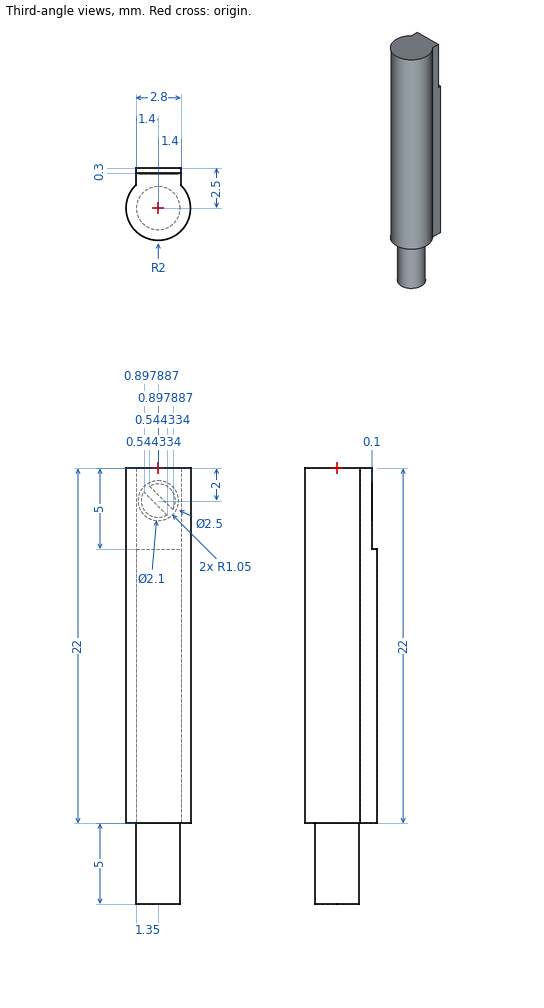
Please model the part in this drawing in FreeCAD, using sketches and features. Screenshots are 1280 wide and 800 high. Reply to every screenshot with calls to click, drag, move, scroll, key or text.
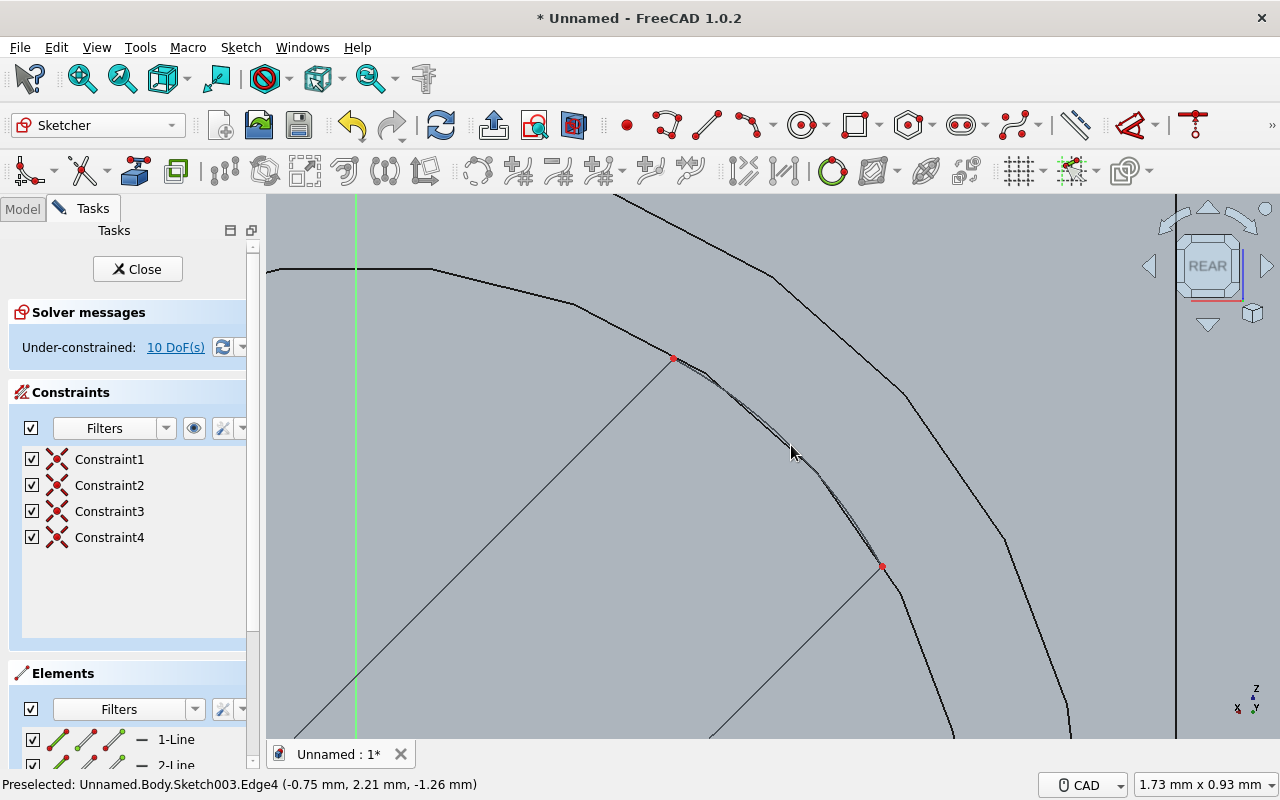
scroll(793, 444, down, 8)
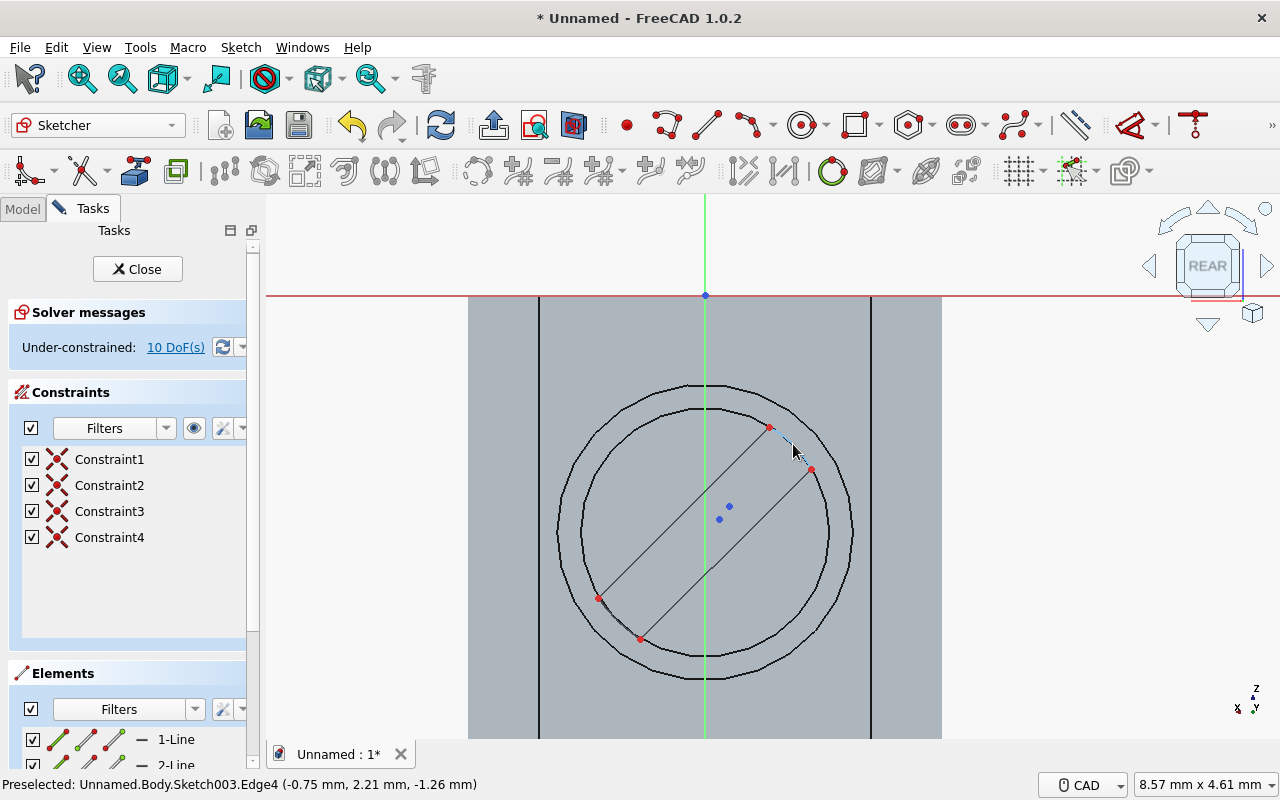
click(609, 612)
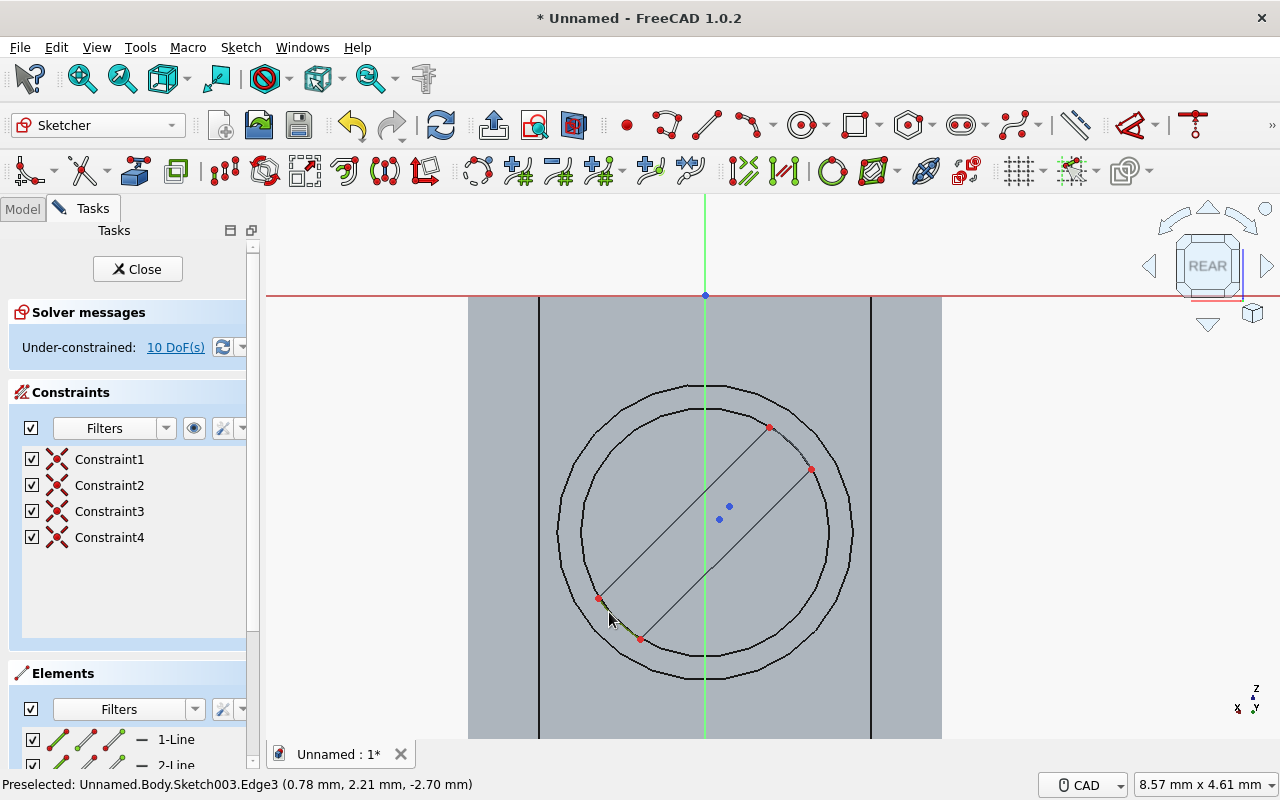
click(801, 454)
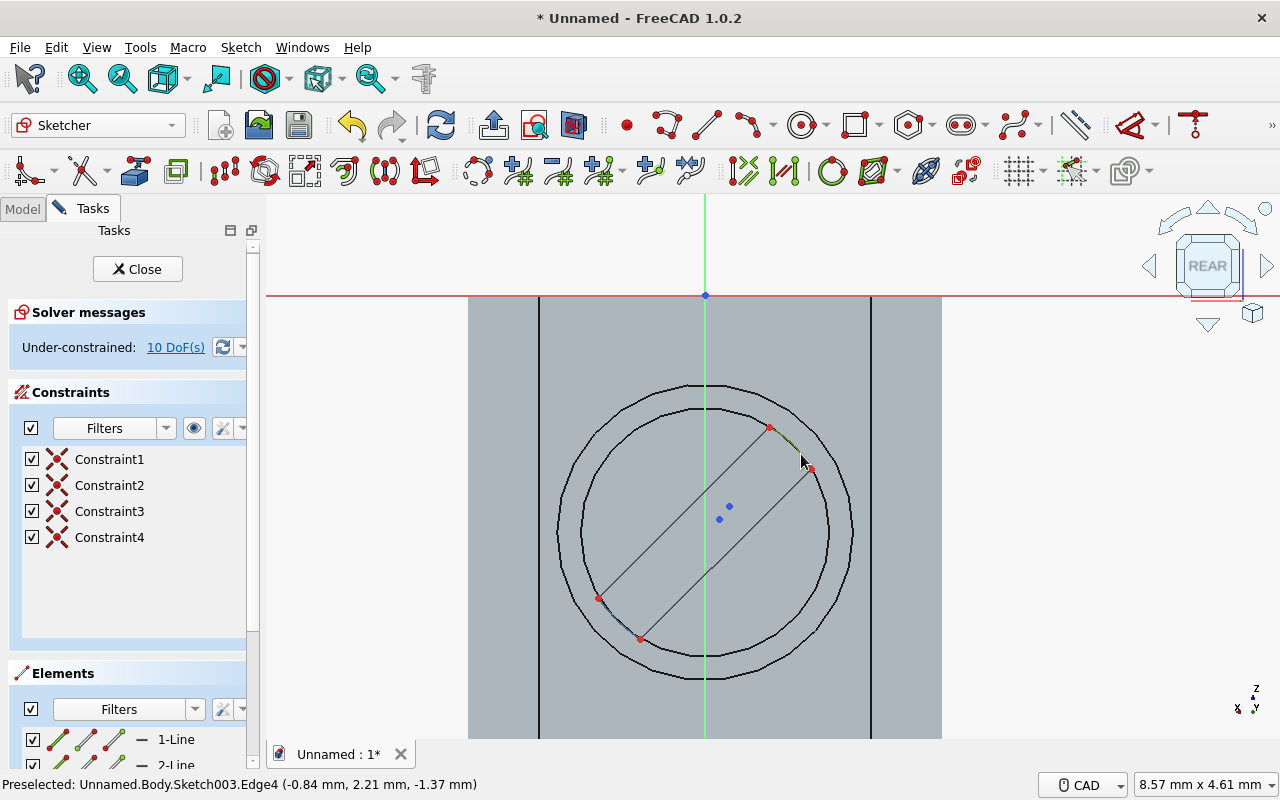
click(1194, 126)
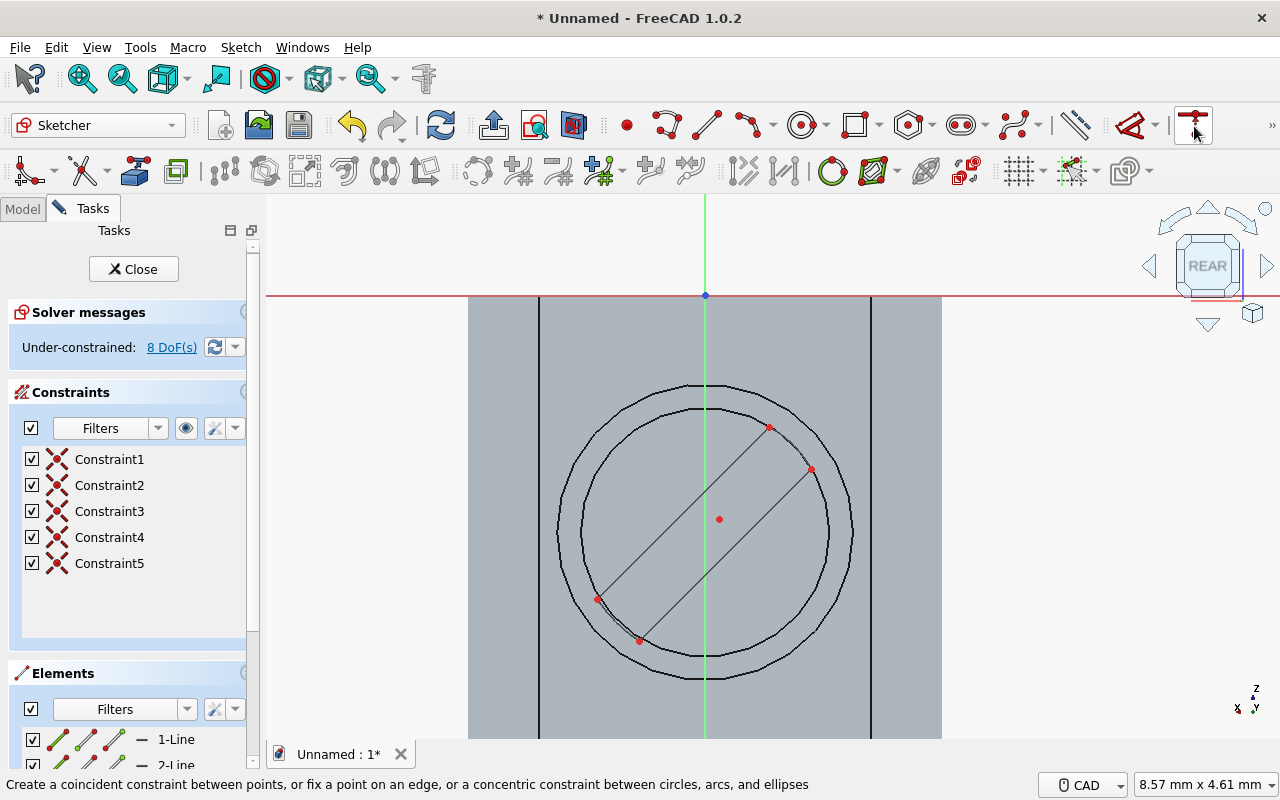
click(608, 614)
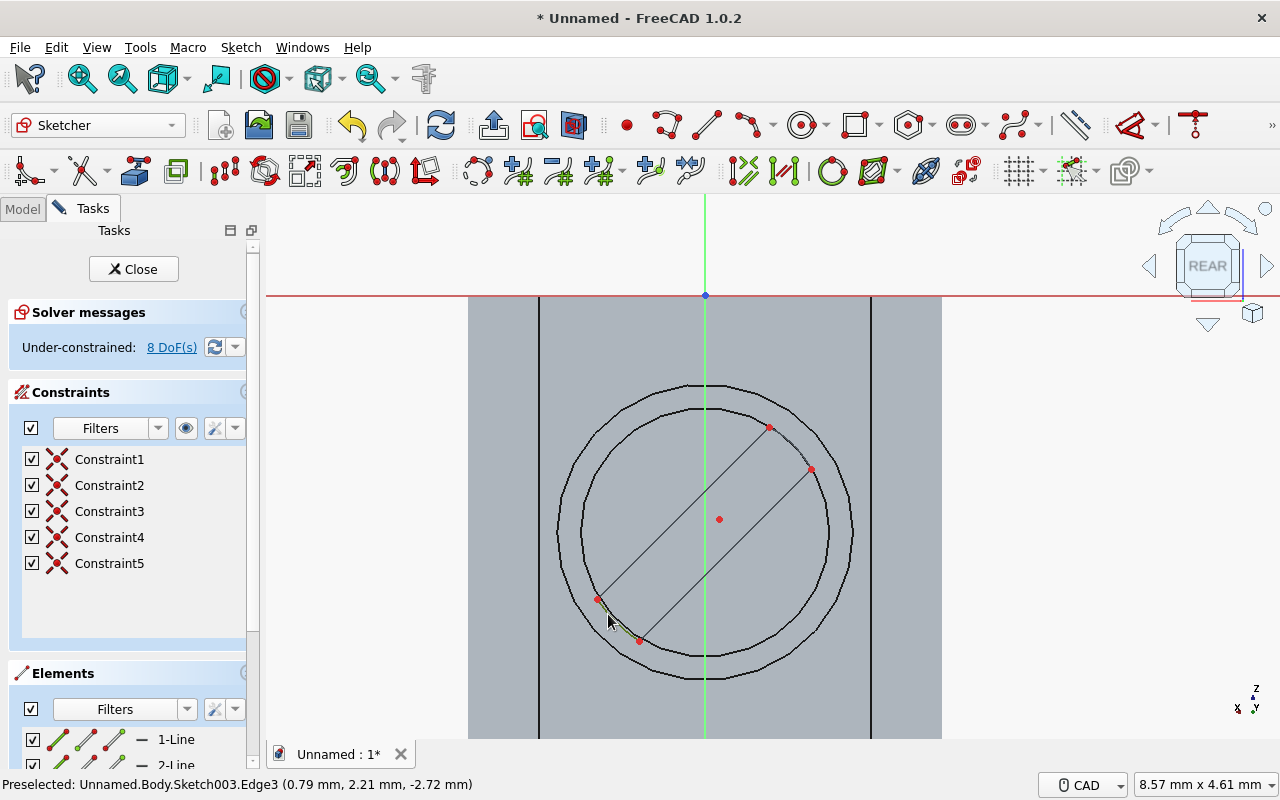
click(801, 454)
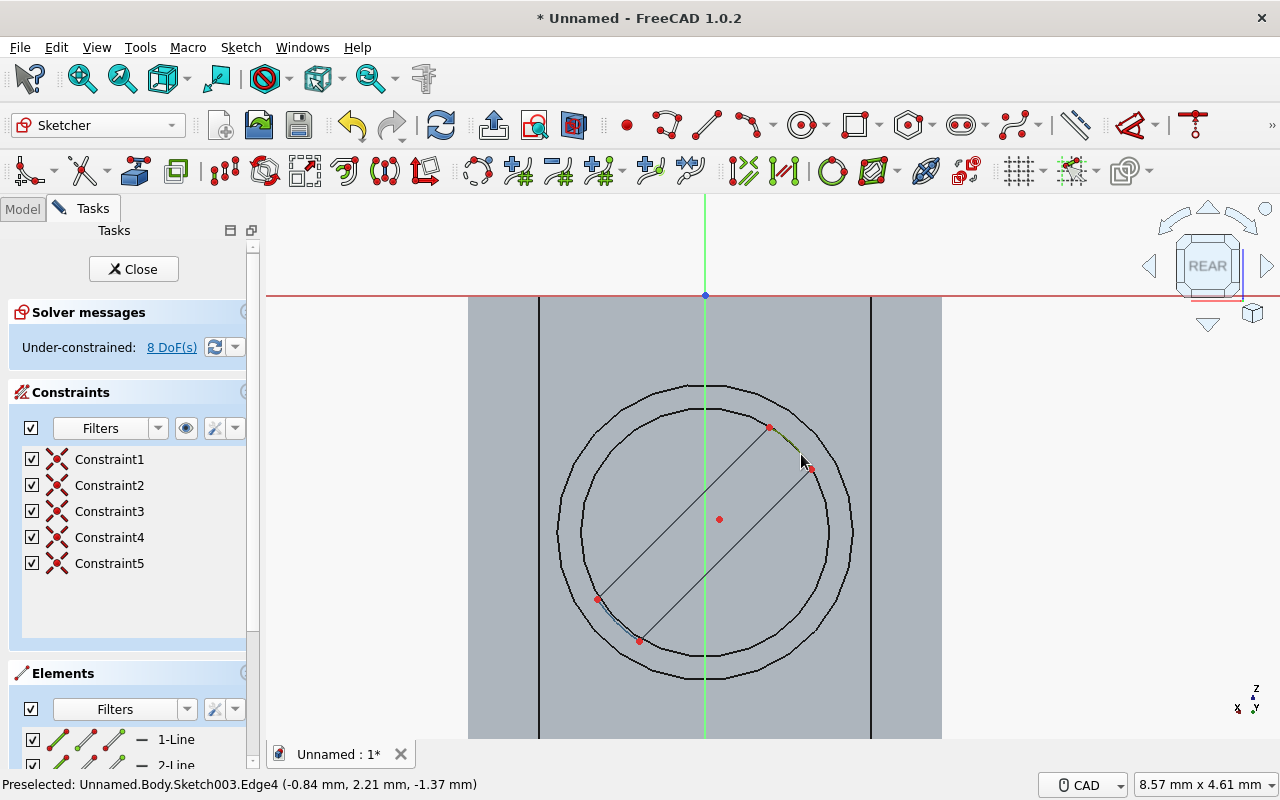
key(e)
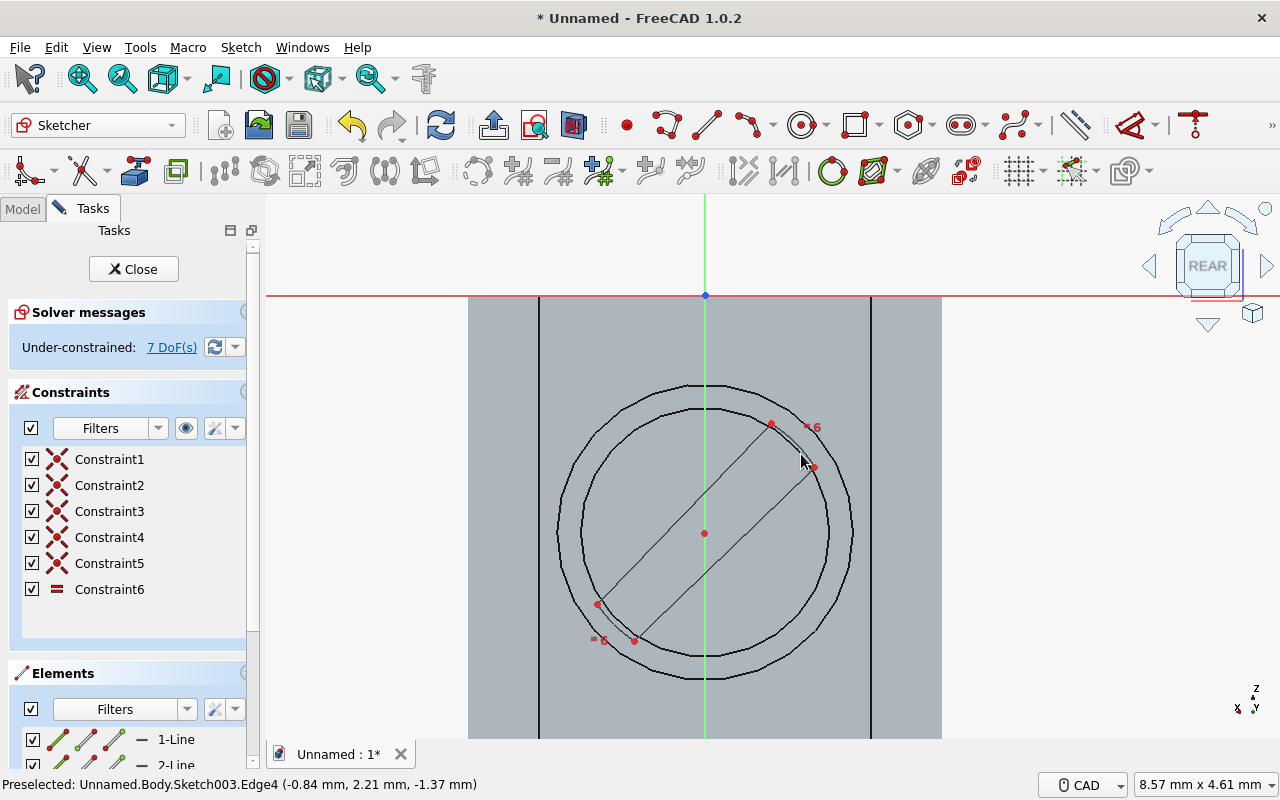
click(705, 534)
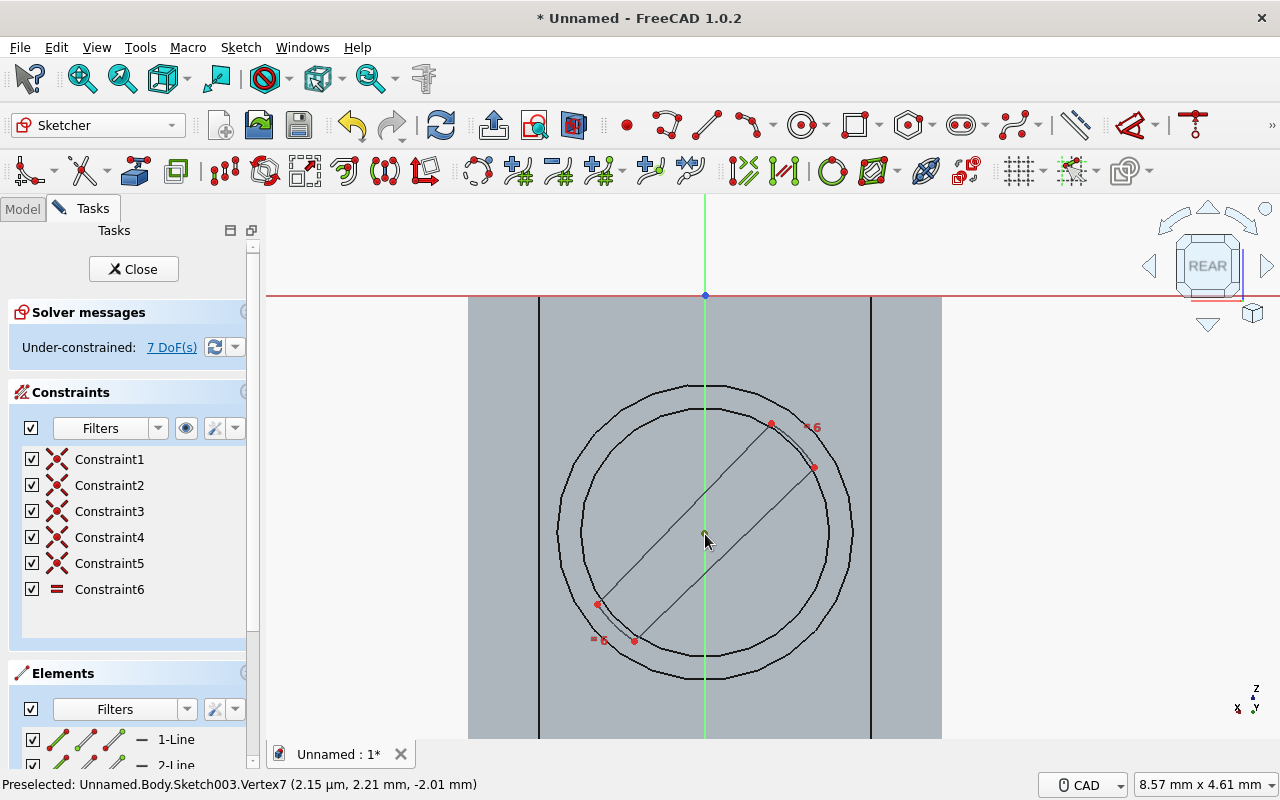
click(705, 676)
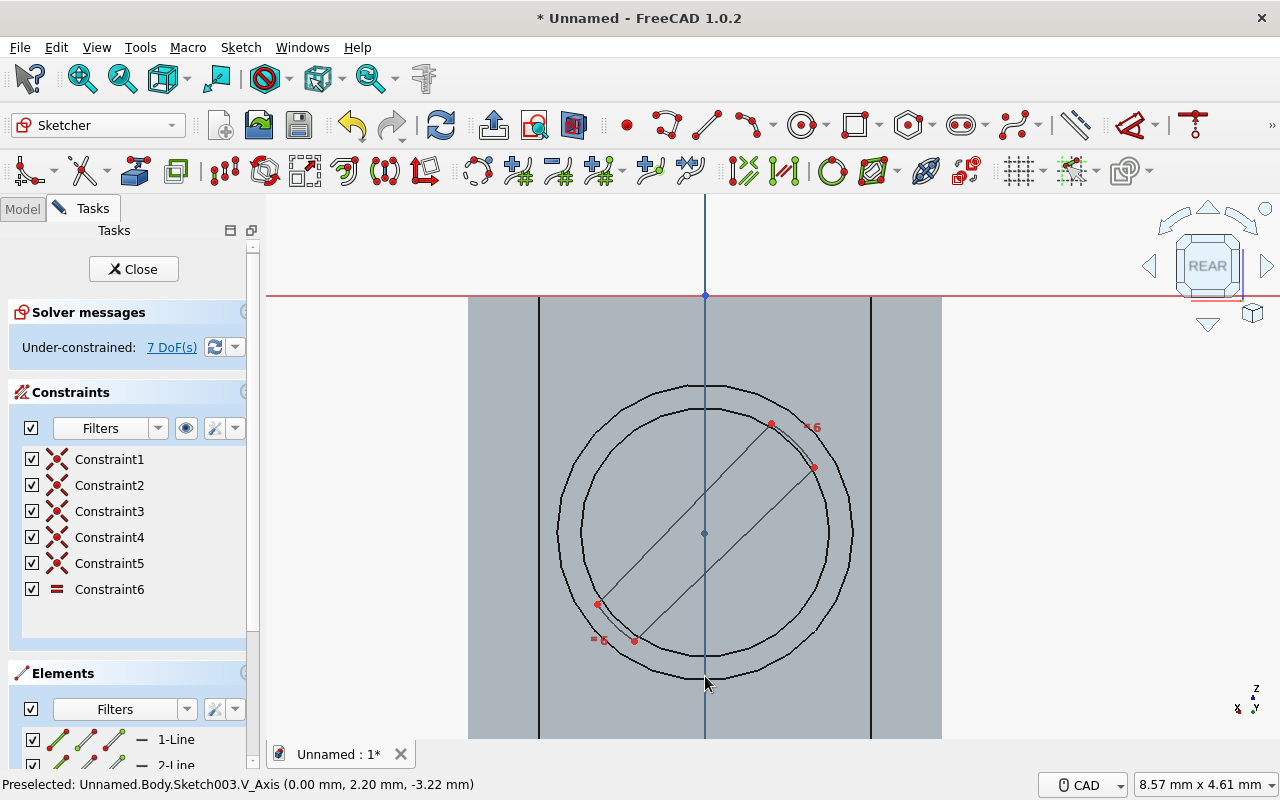
click(1194, 126)